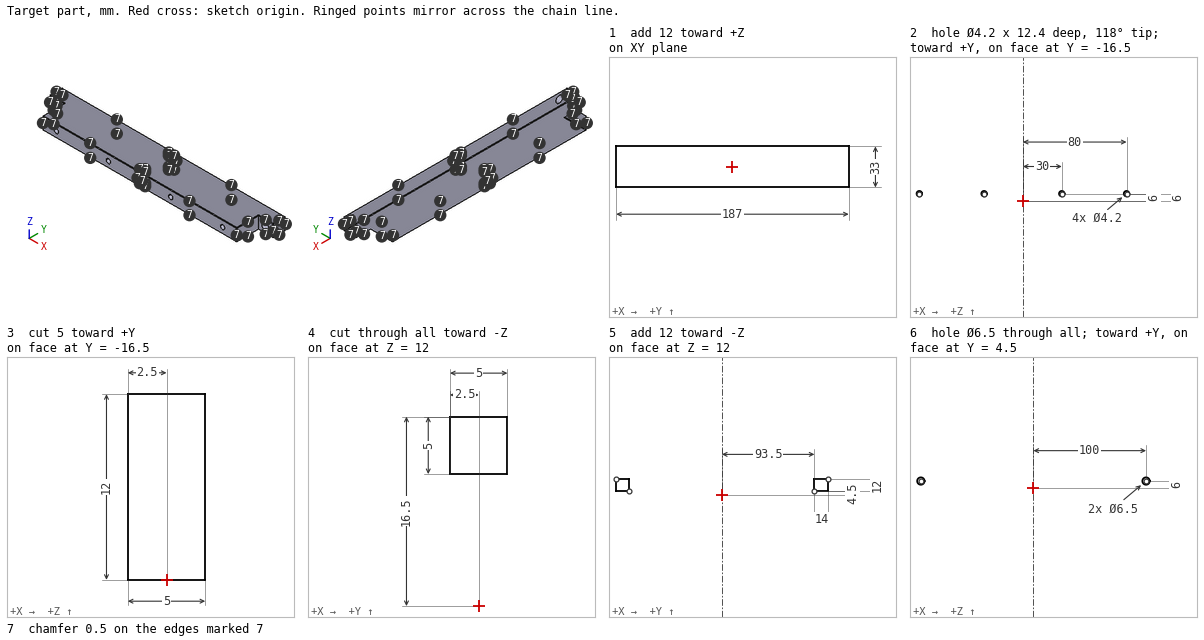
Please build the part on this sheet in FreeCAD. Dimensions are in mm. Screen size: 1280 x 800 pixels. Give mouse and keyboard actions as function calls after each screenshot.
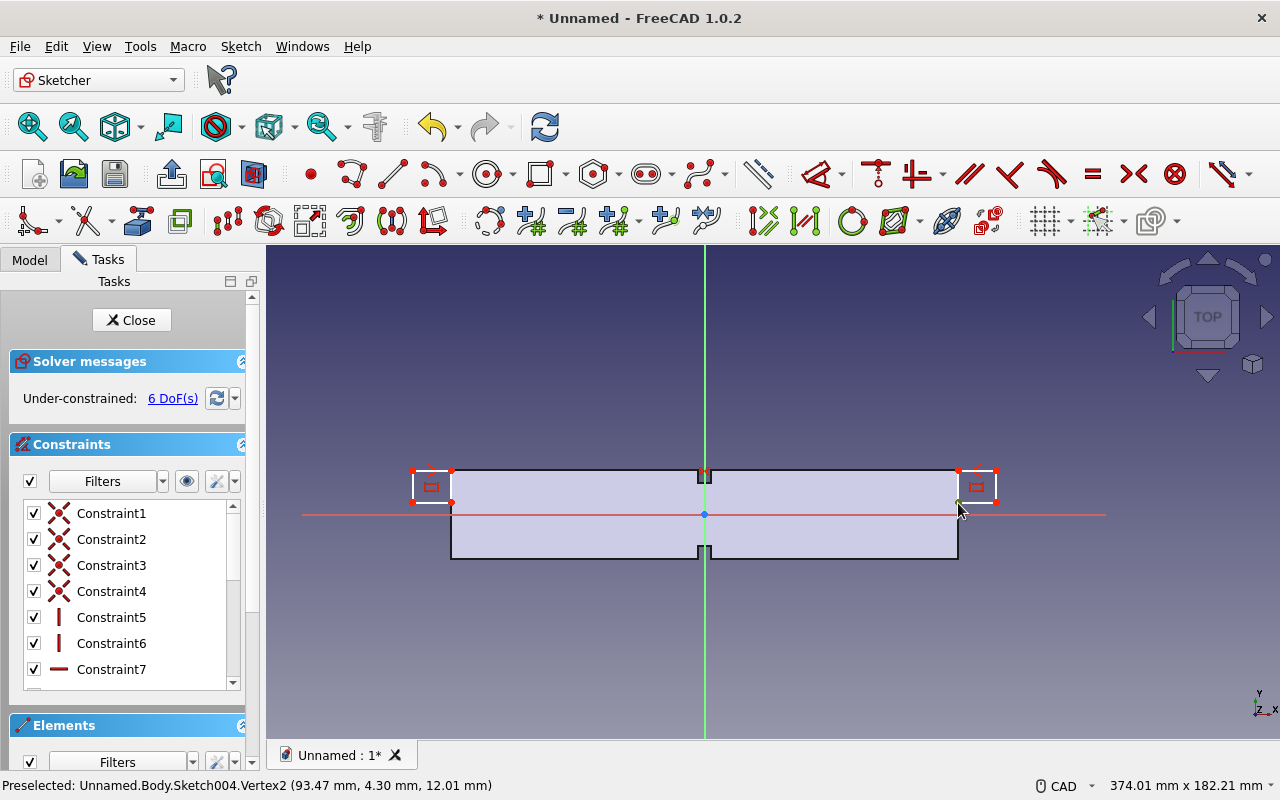
click(451, 503)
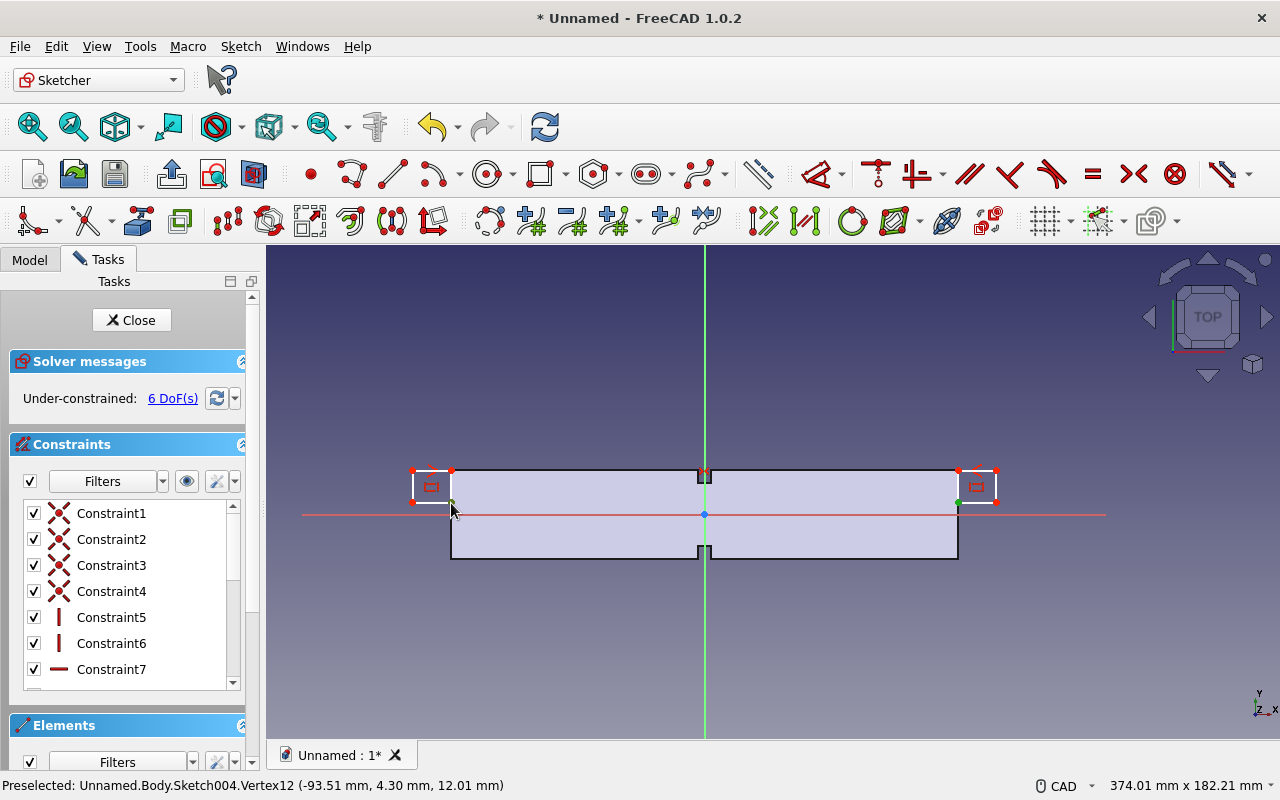
click(705, 680)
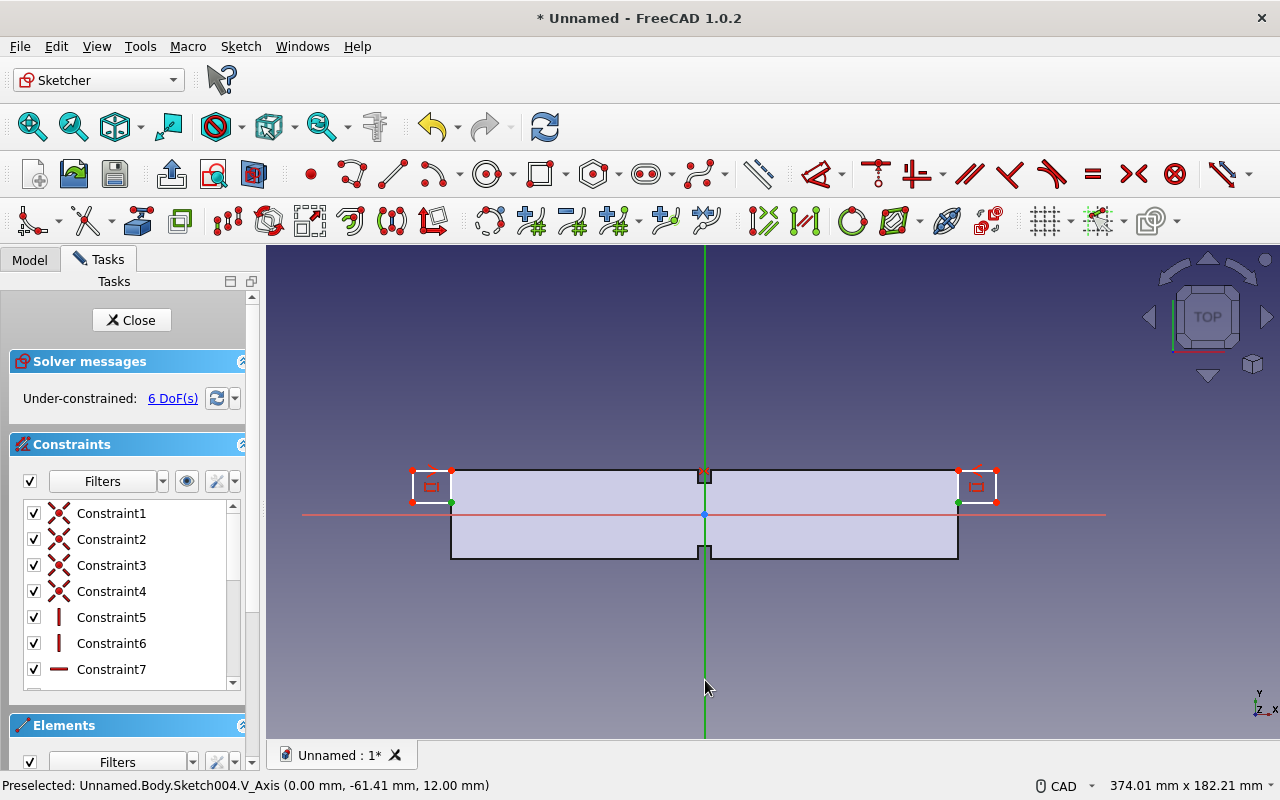
click(1134, 174)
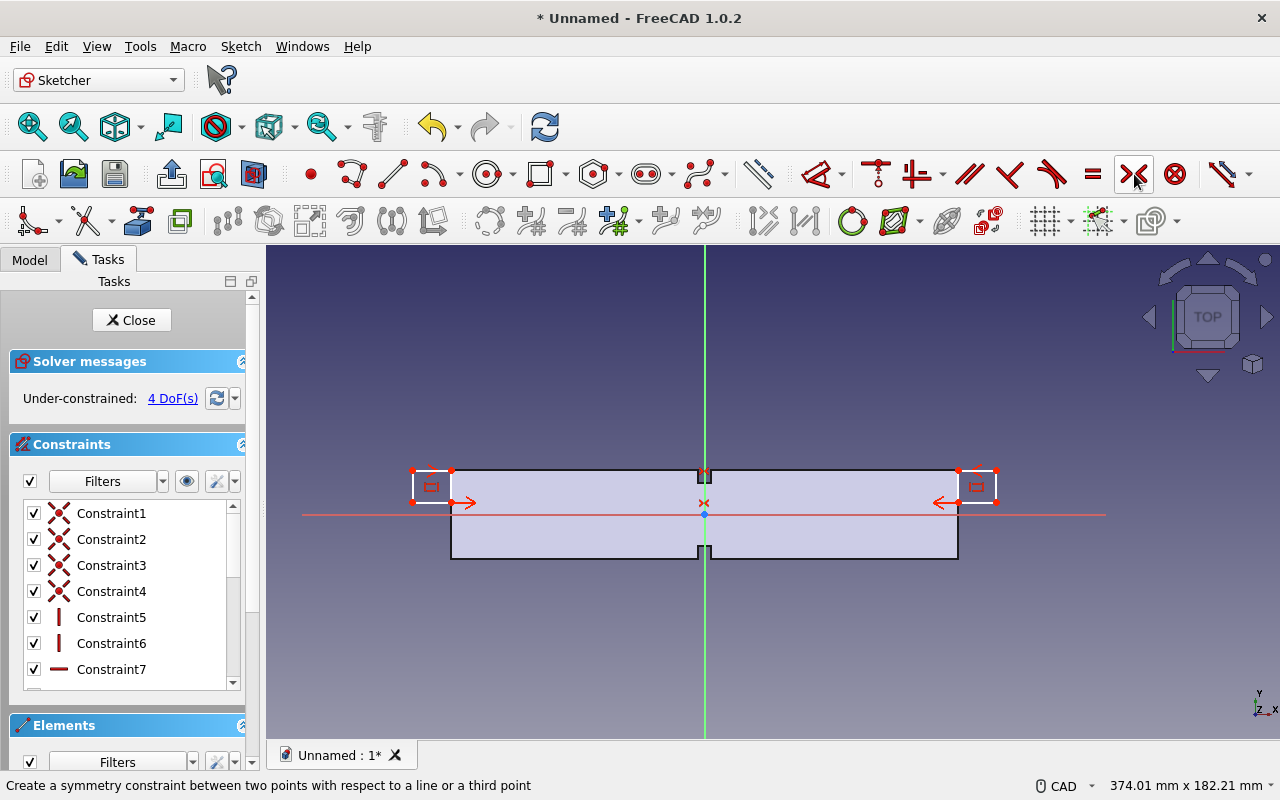
key(d)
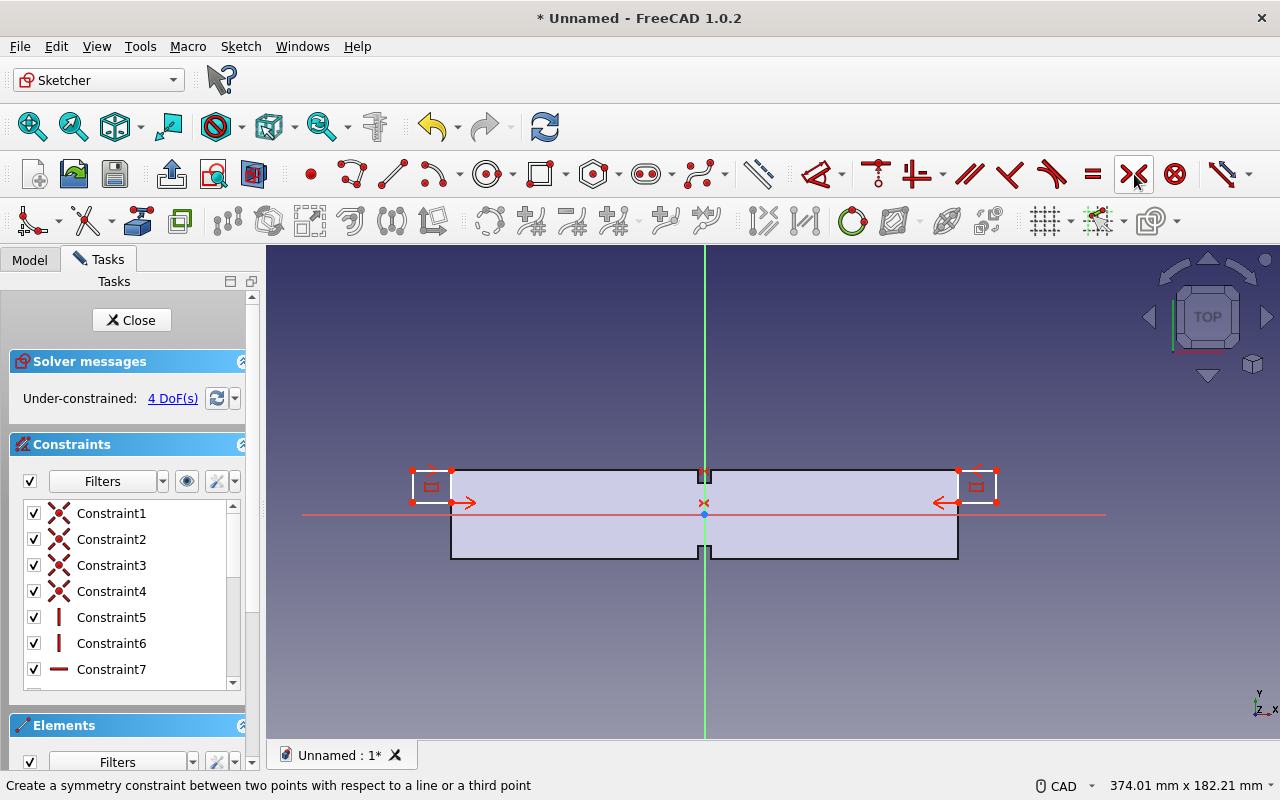
scroll(958, 480, up, 2)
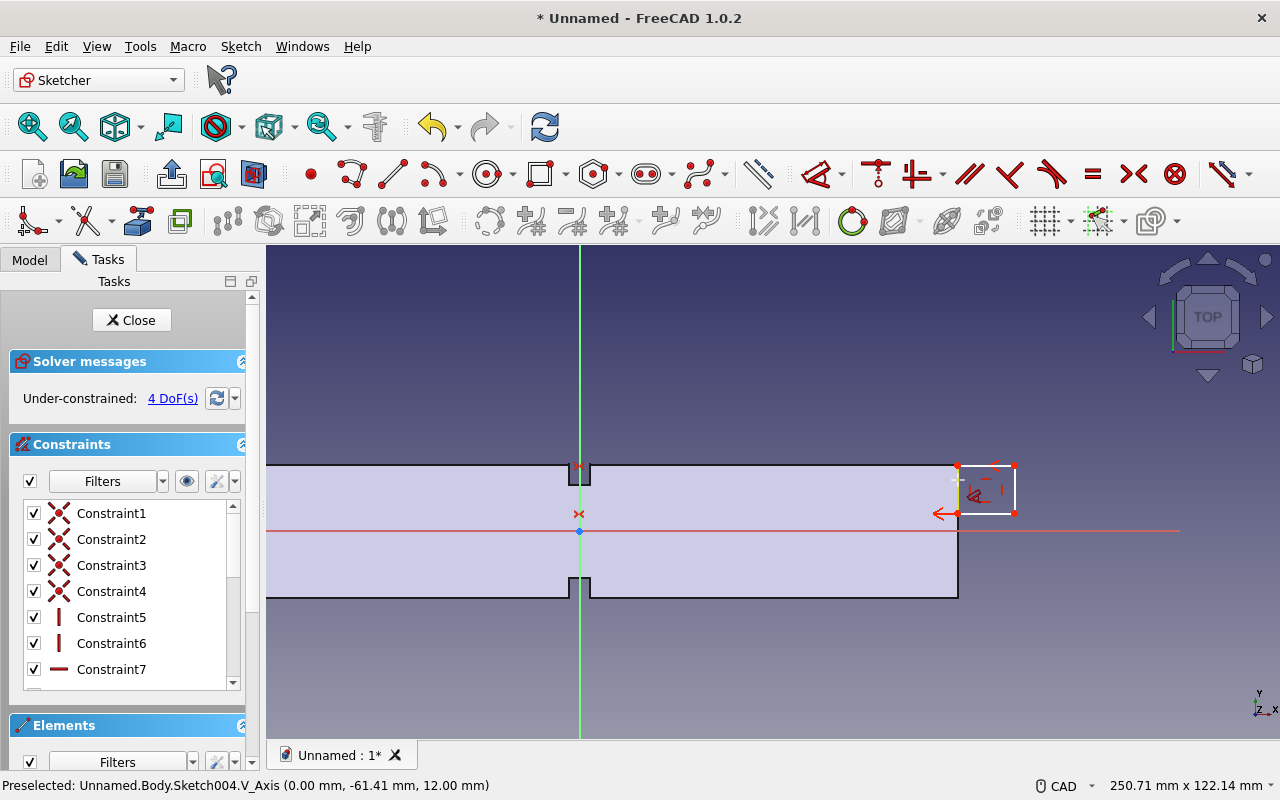
click(958, 480)
click(992, 490)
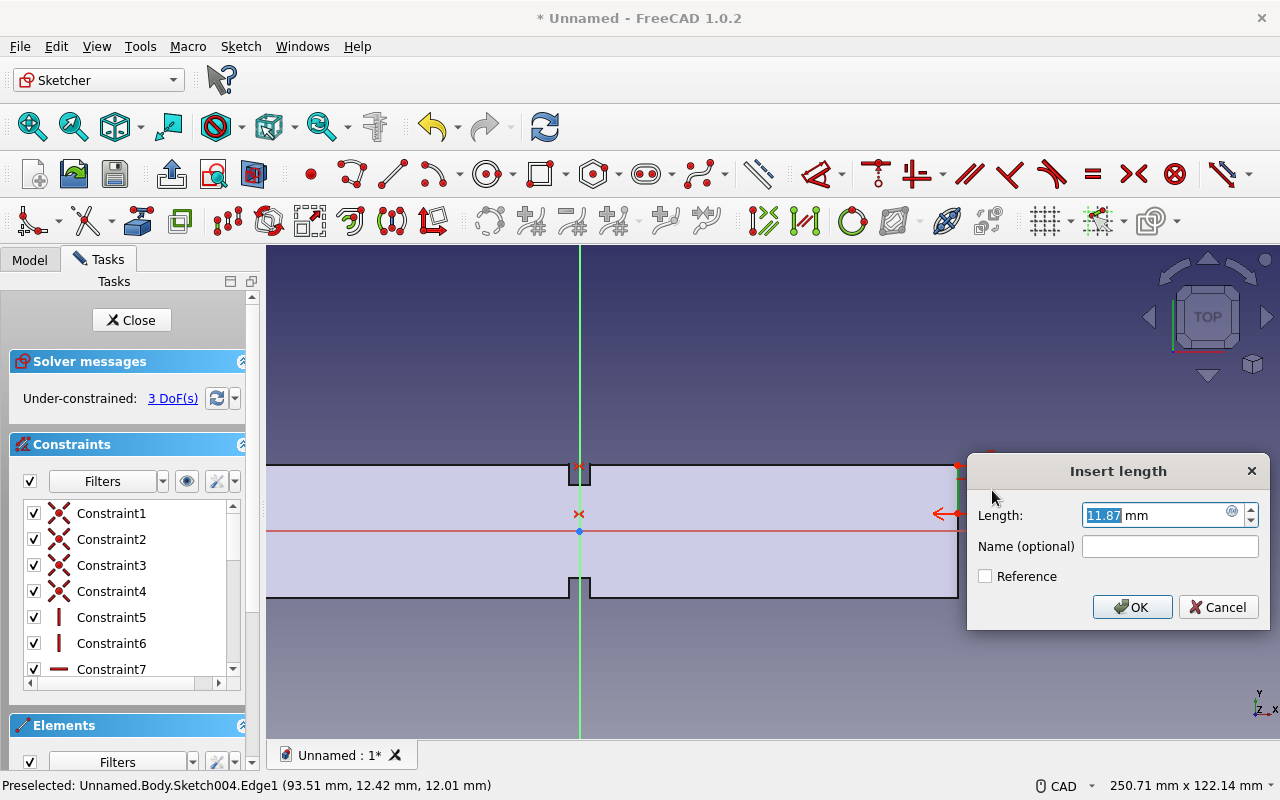
text(12)
key(Return)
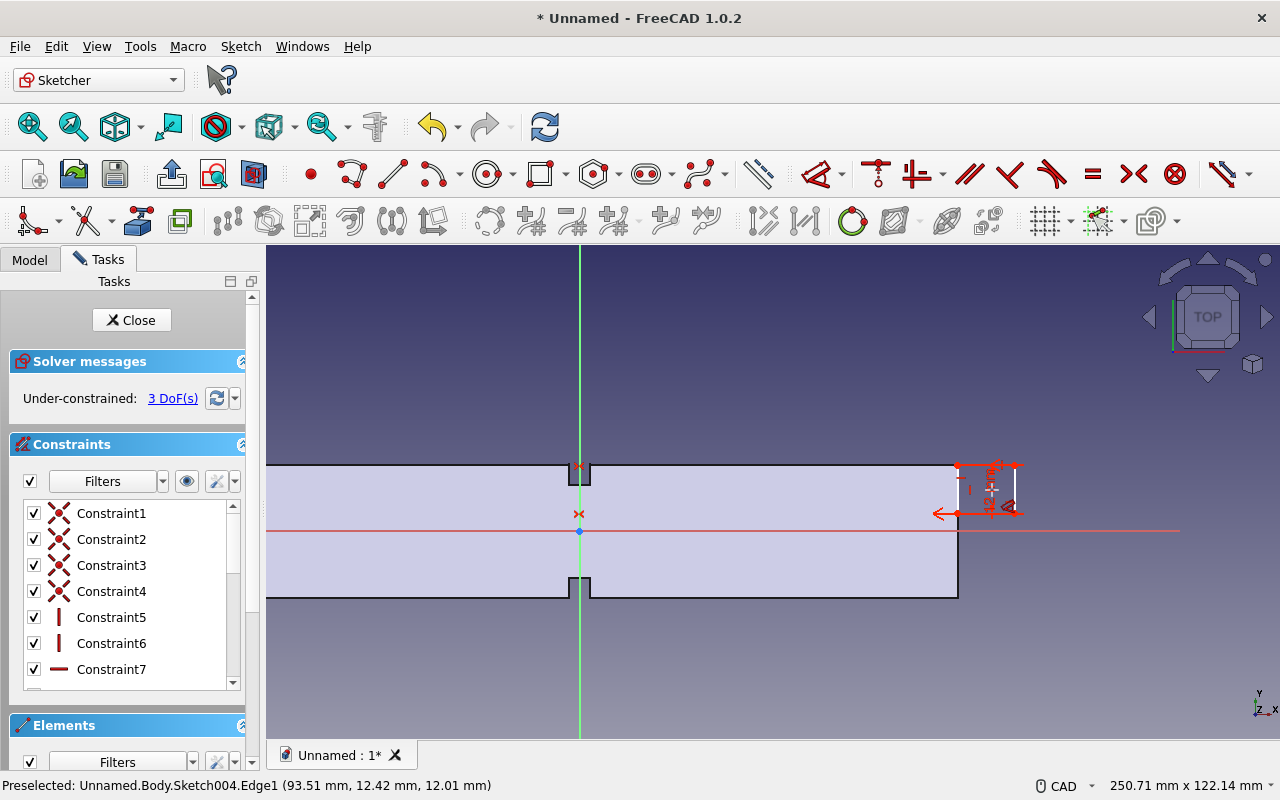
click(975, 514)
click(986, 548)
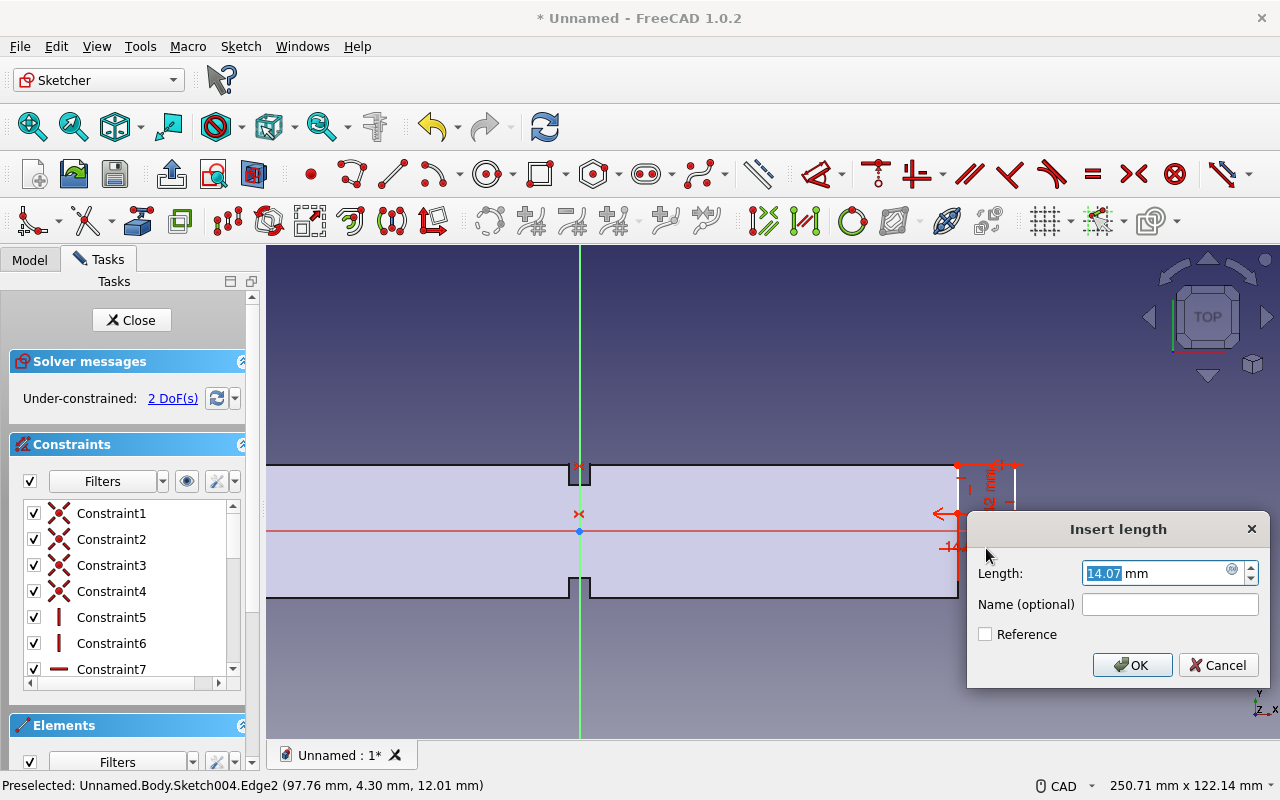
text(14)
key(Return)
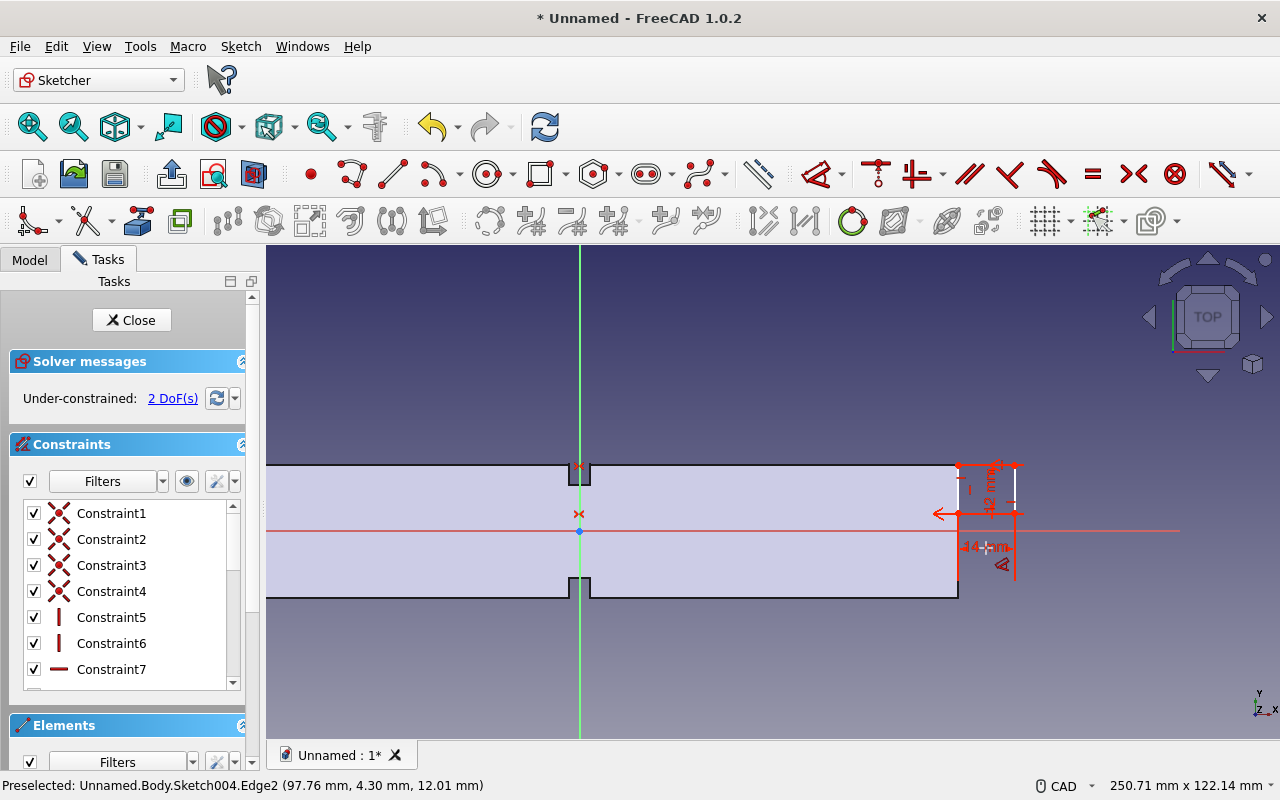
scroll(958, 514, up, 4)